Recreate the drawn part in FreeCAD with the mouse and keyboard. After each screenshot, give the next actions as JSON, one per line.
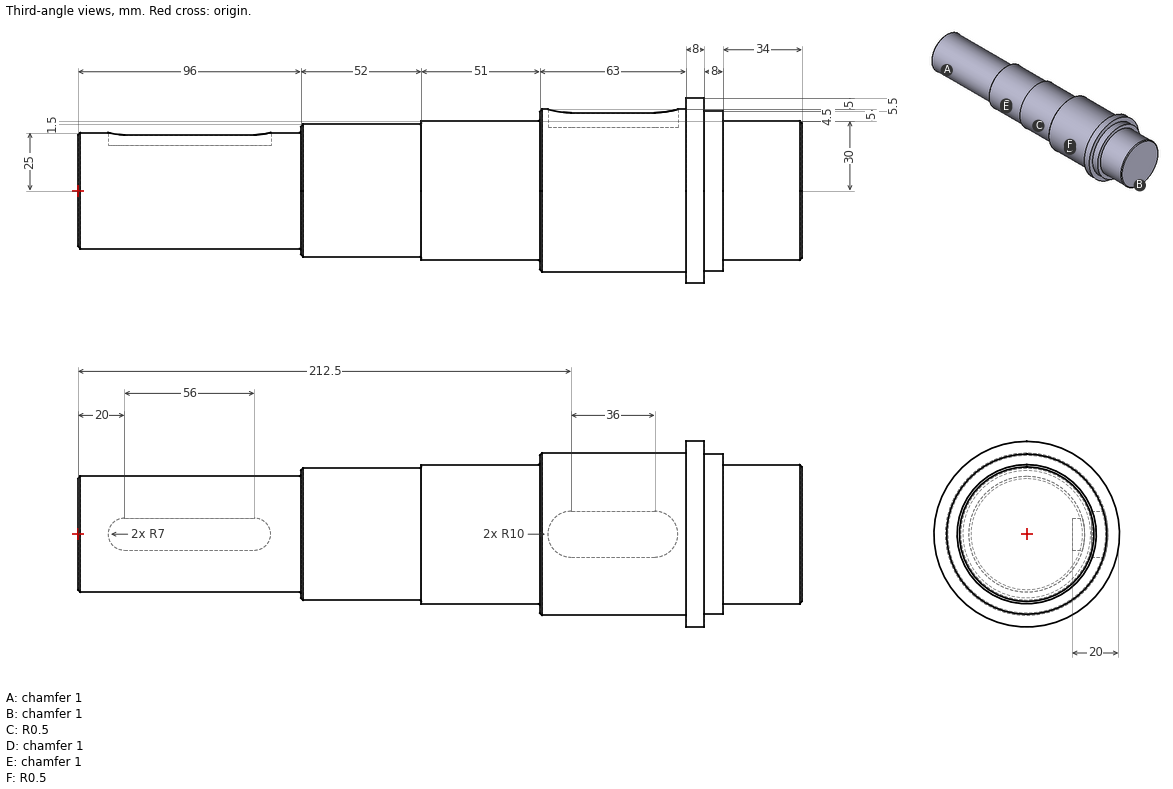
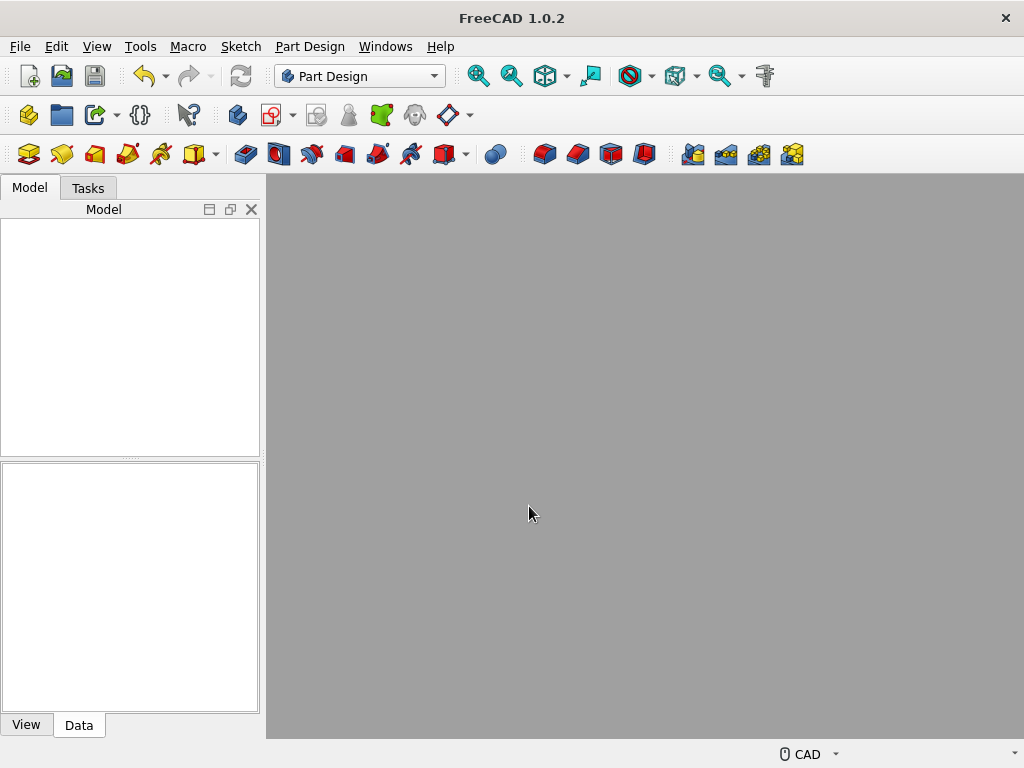
{"action": "key", "text": "ctrl+n"}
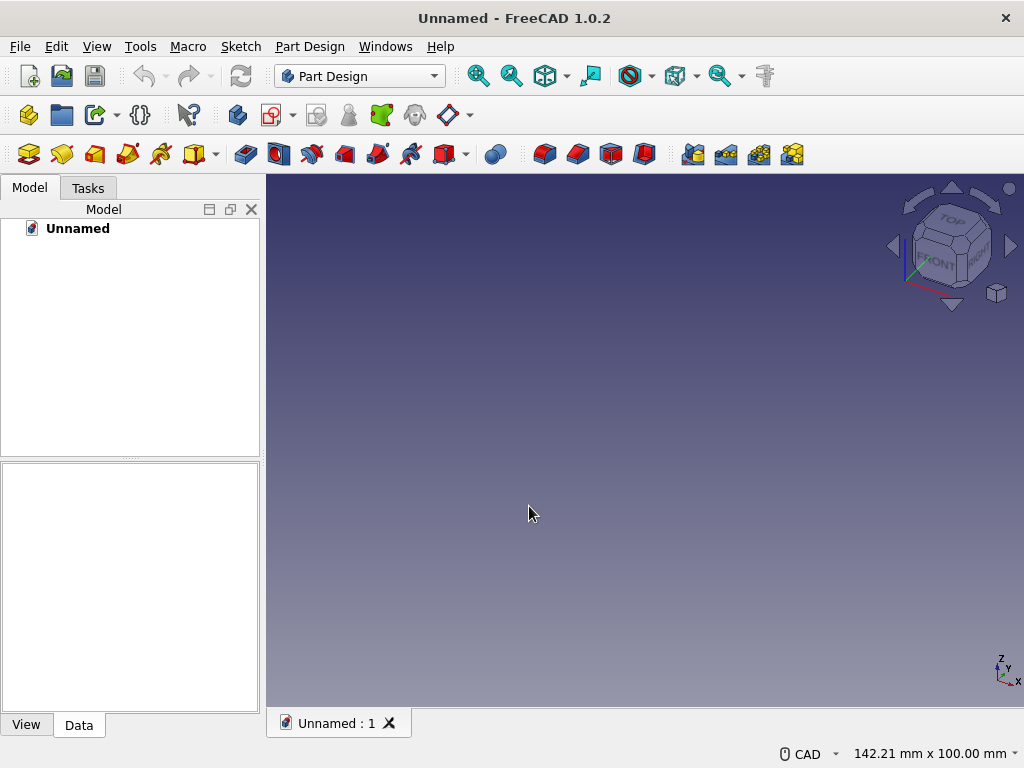
{"action": "left_click", "coordinate": [270, 116]}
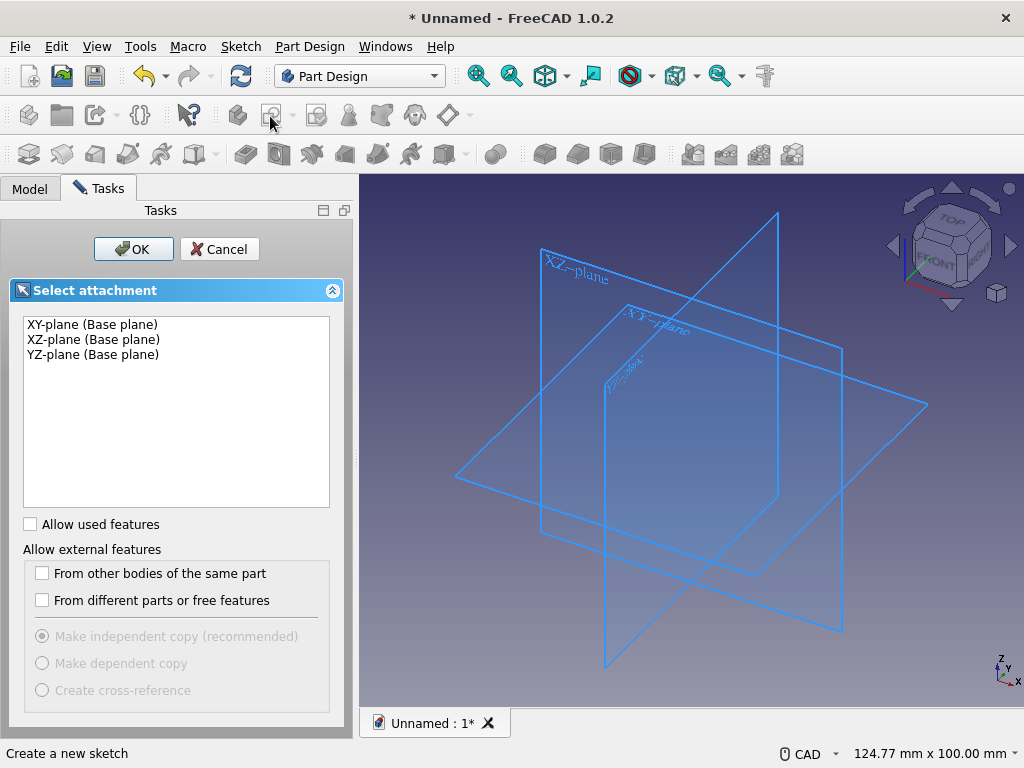
{"action": "left_click", "coordinate": [84, 324]}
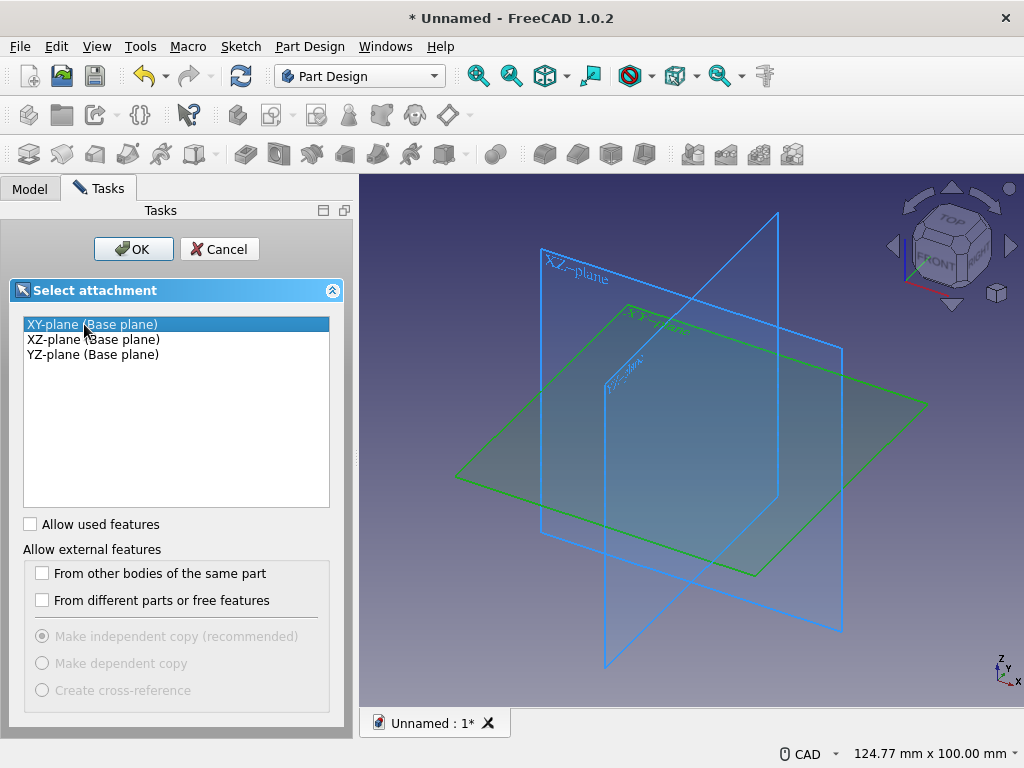
{"action": "left_click", "coordinate": [134, 249]}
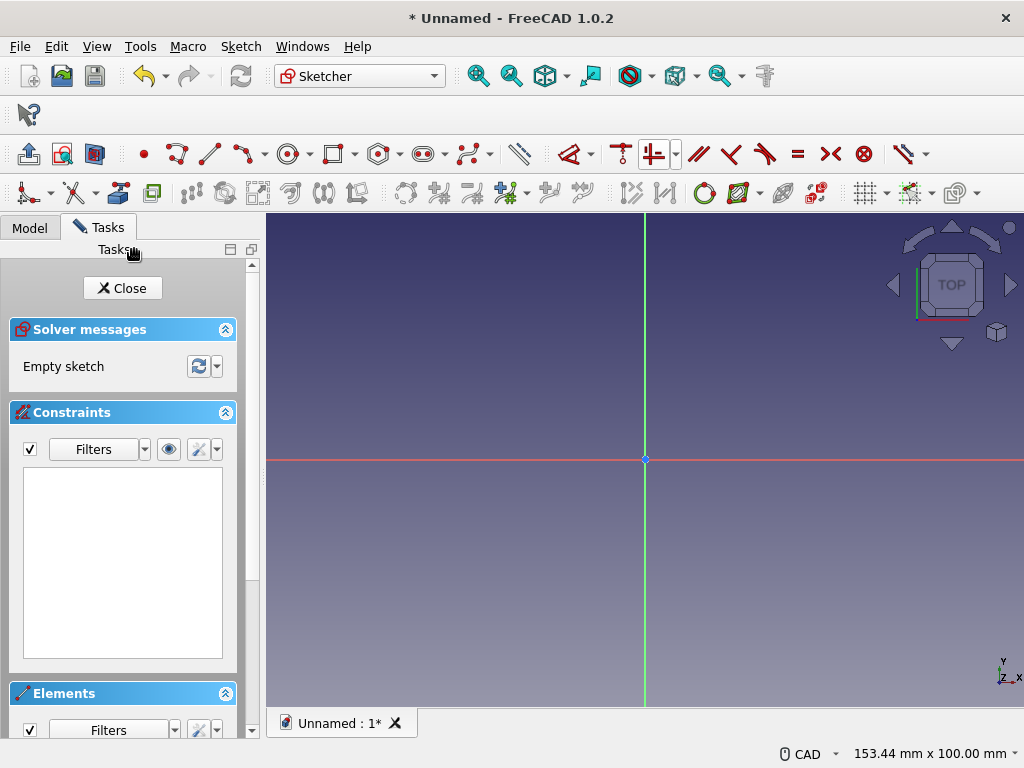
{"action": "scroll", "coordinate": [302, 492], "scroll_direction": "down", "scroll_amount": 7}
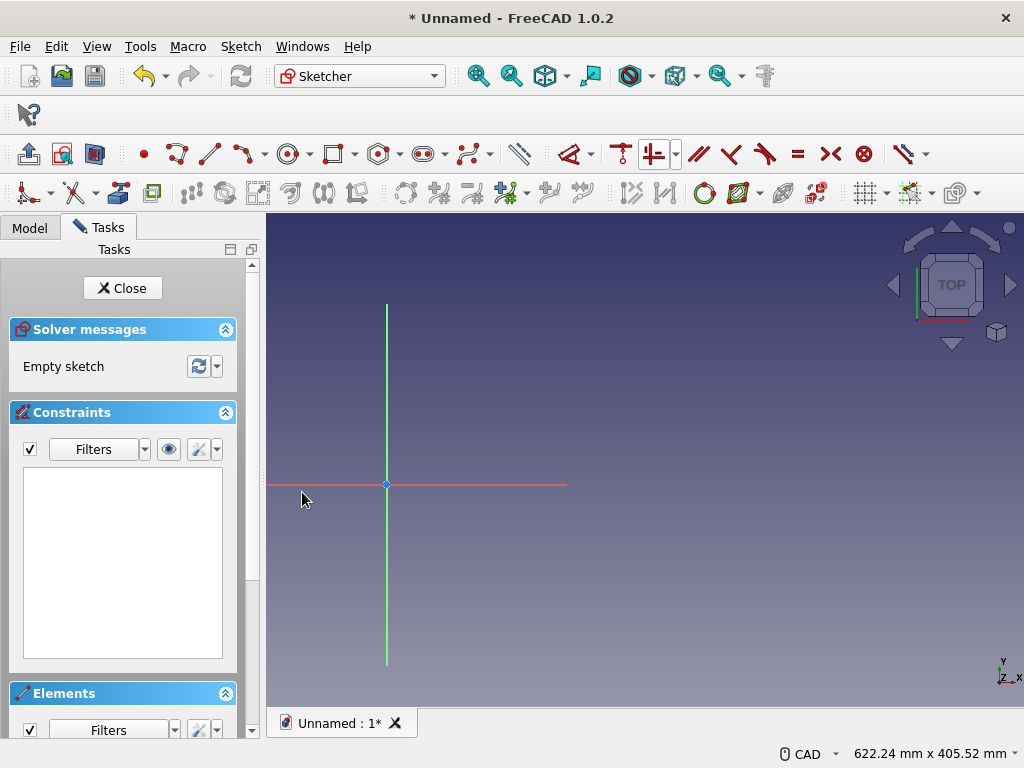
{"action": "key", "text": "g m"}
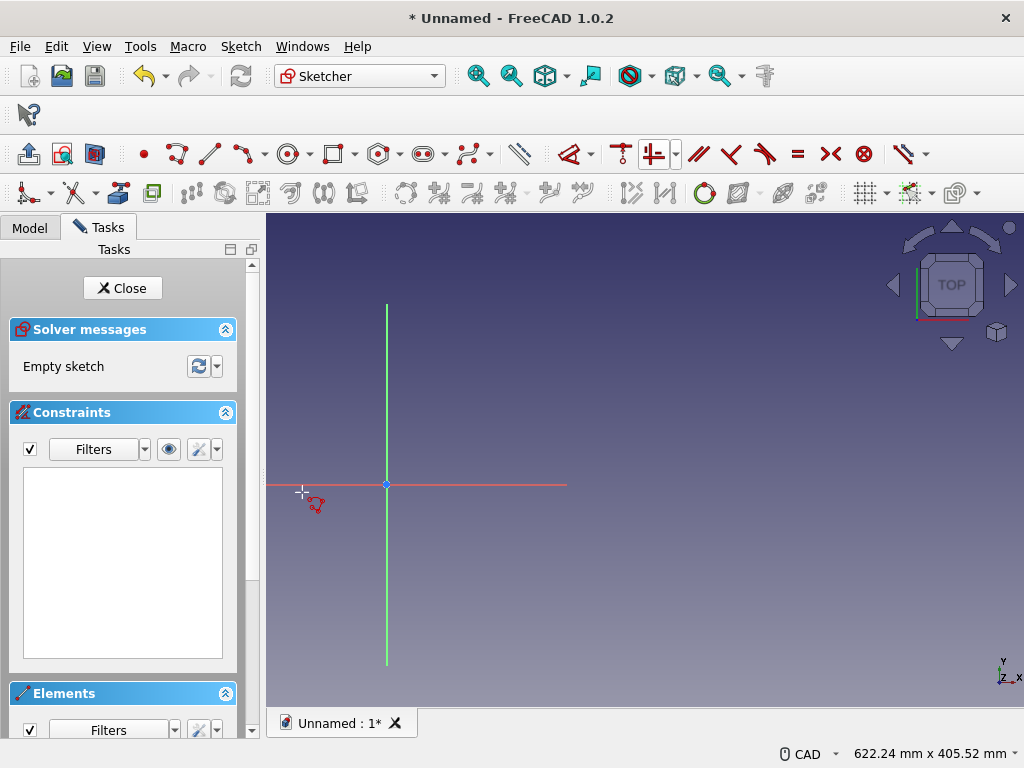
{"action": "left_click", "coordinate": [387, 485]}
{"action": "left_click", "coordinate": [767, 476]}
{"action": "left_click", "coordinate": [767, 448]}
{"action": "left_click", "coordinate": [725, 448]}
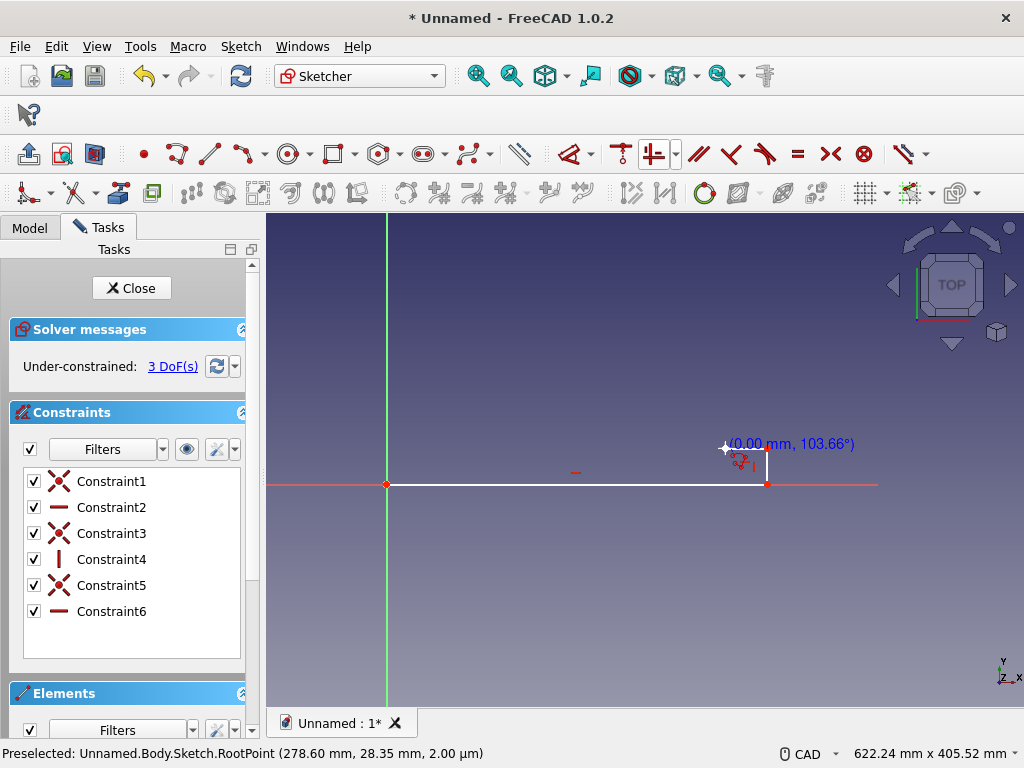
{"action": "scroll", "coordinate": [725, 443], "scroll_direction": "up", "scroll_amount": 6}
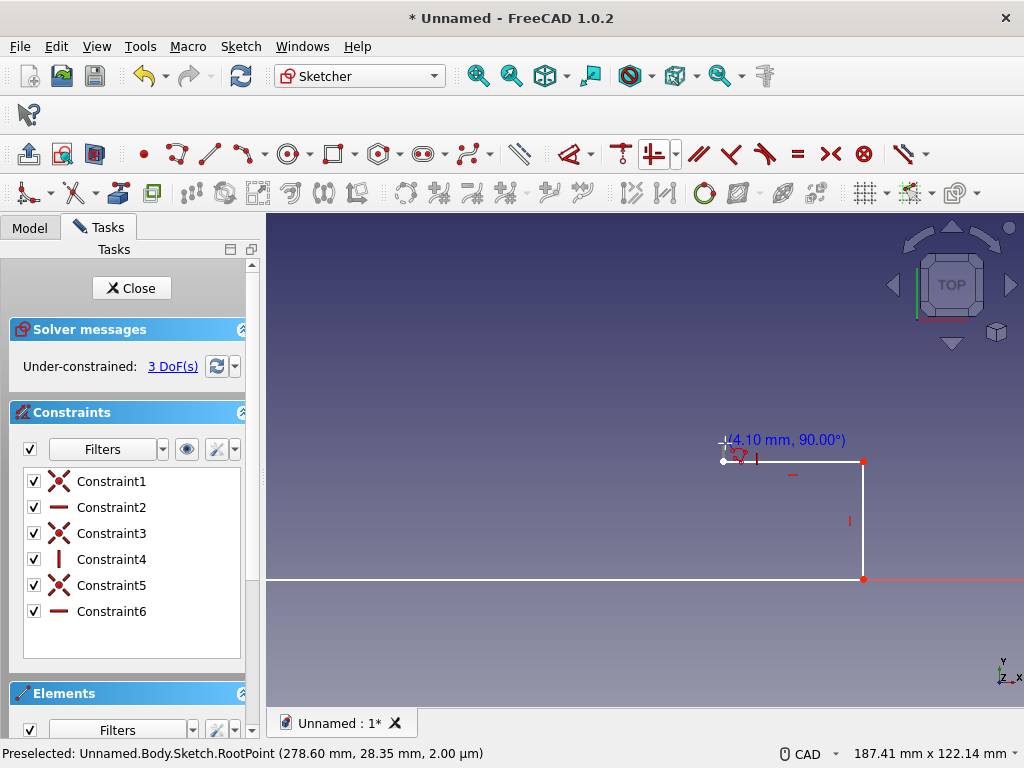
{"action": "left_click", "coordinate": [724, 440]}
{"action": "left_click", "coordinate": [692, 440]}
{"action": "left_click", "coordinate": [692, 418]}
{"action": "left_click", "coordinate": [660, 418]}
{"action": "left_click", "coordinate": [660, 438]}
{"action": "left_click", "coordinate": [405, 438]}
{"action": "left_click", "coordinate": [405, 458]}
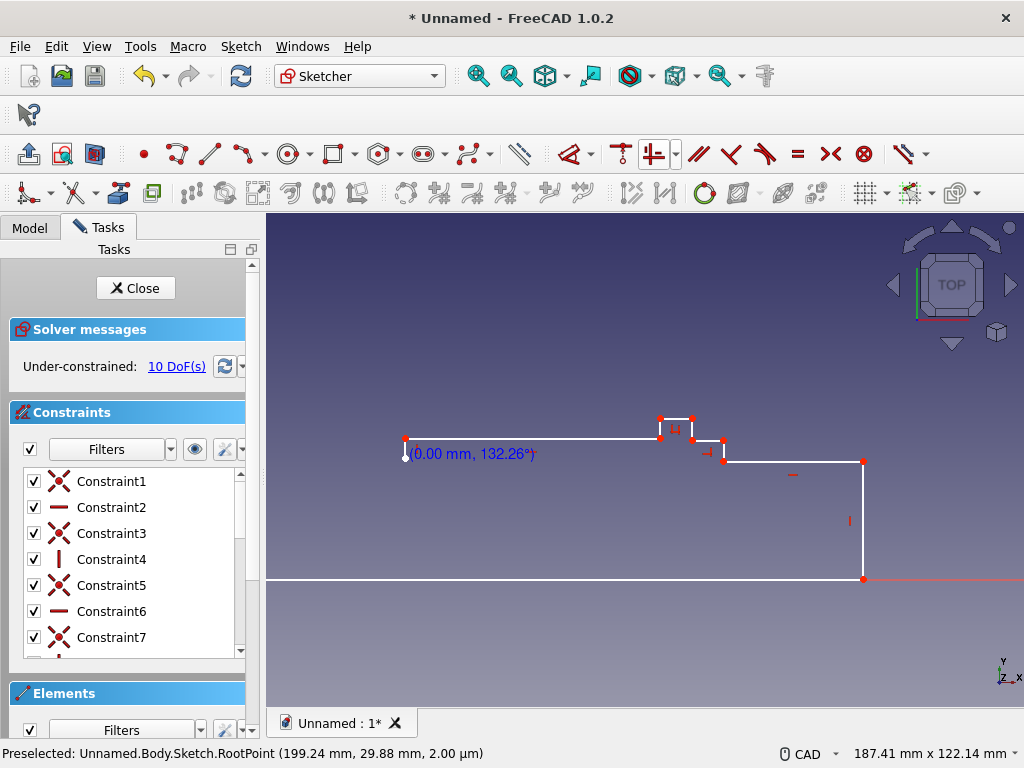
{"action": "scroll", "coordinate": [725, 443], "scroll_direction": "down", "scroll_amount": 6}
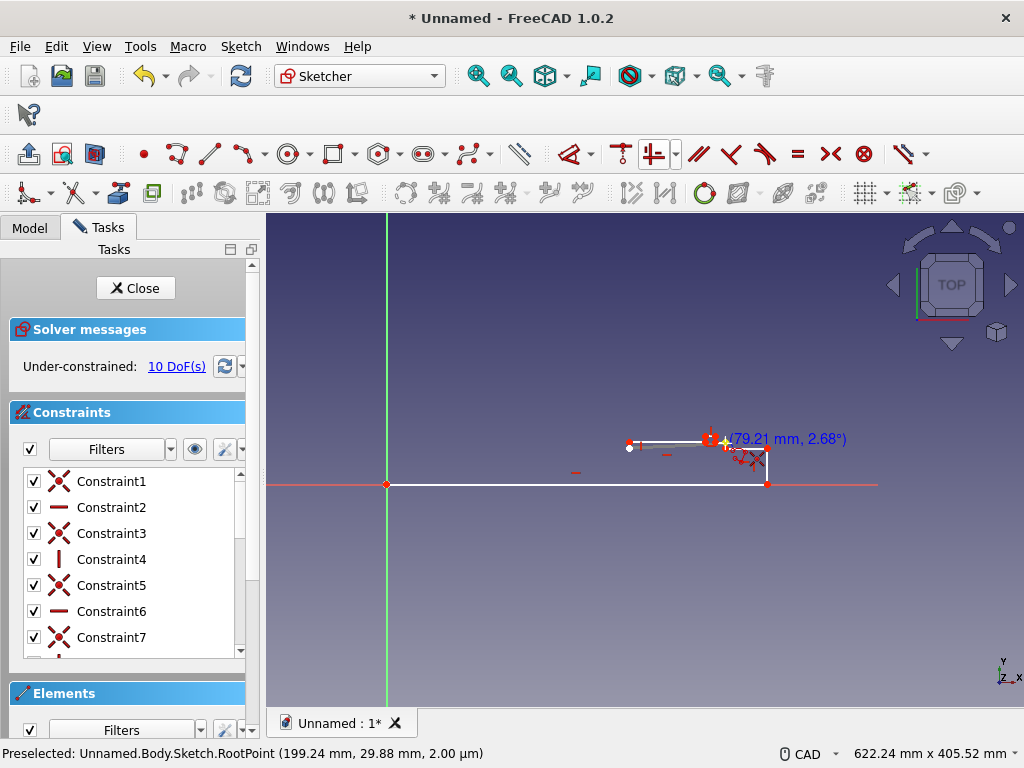
{"action": "left_click", "coordinate": [567, 448]}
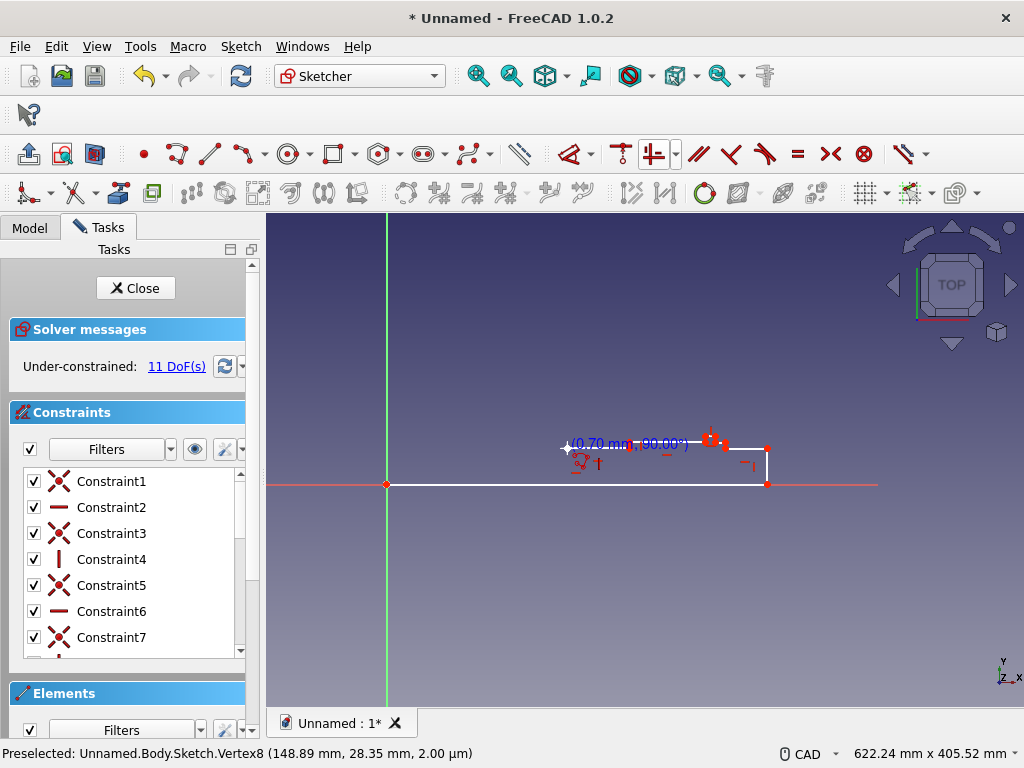
{"action": "scroll", "coordinate": [567, 450], "scroll_direction": "up", "scroll_amount": 11}